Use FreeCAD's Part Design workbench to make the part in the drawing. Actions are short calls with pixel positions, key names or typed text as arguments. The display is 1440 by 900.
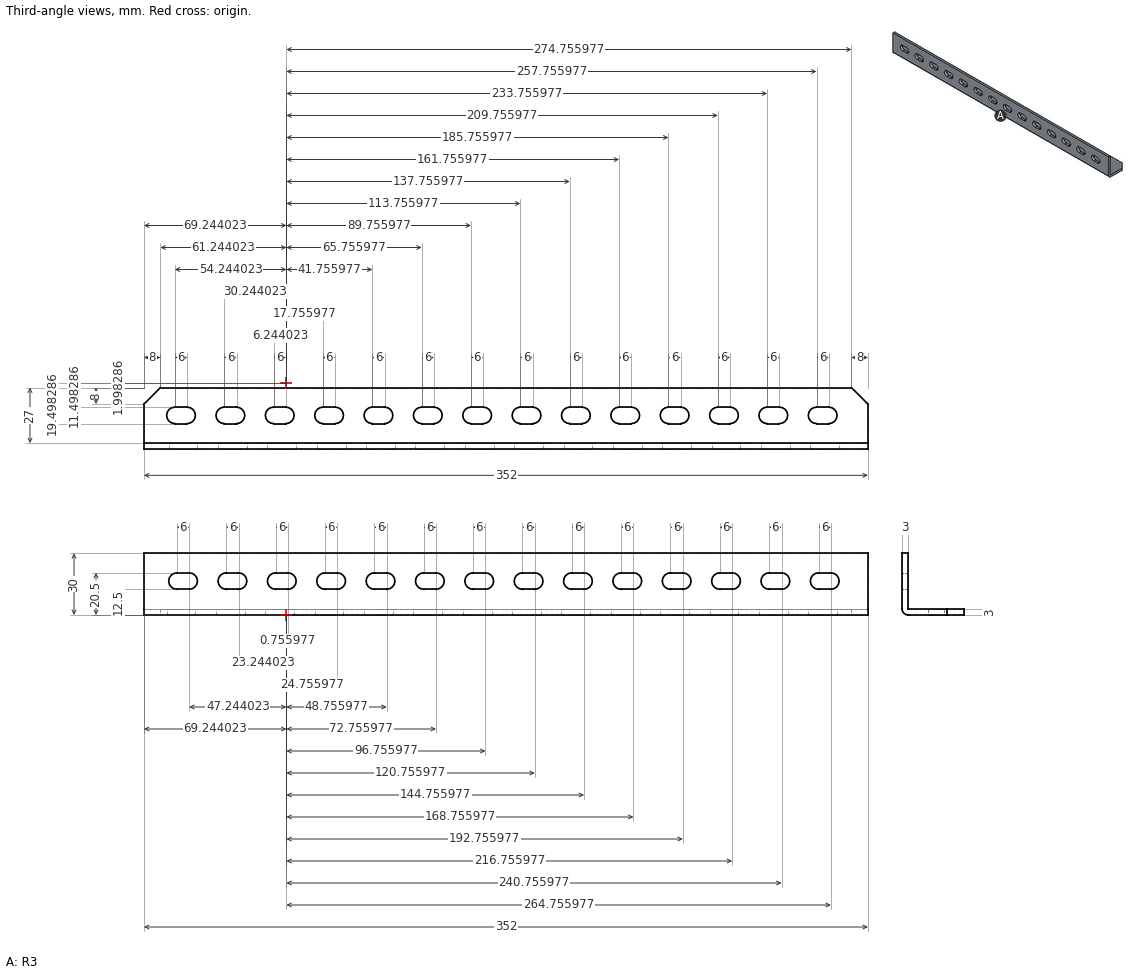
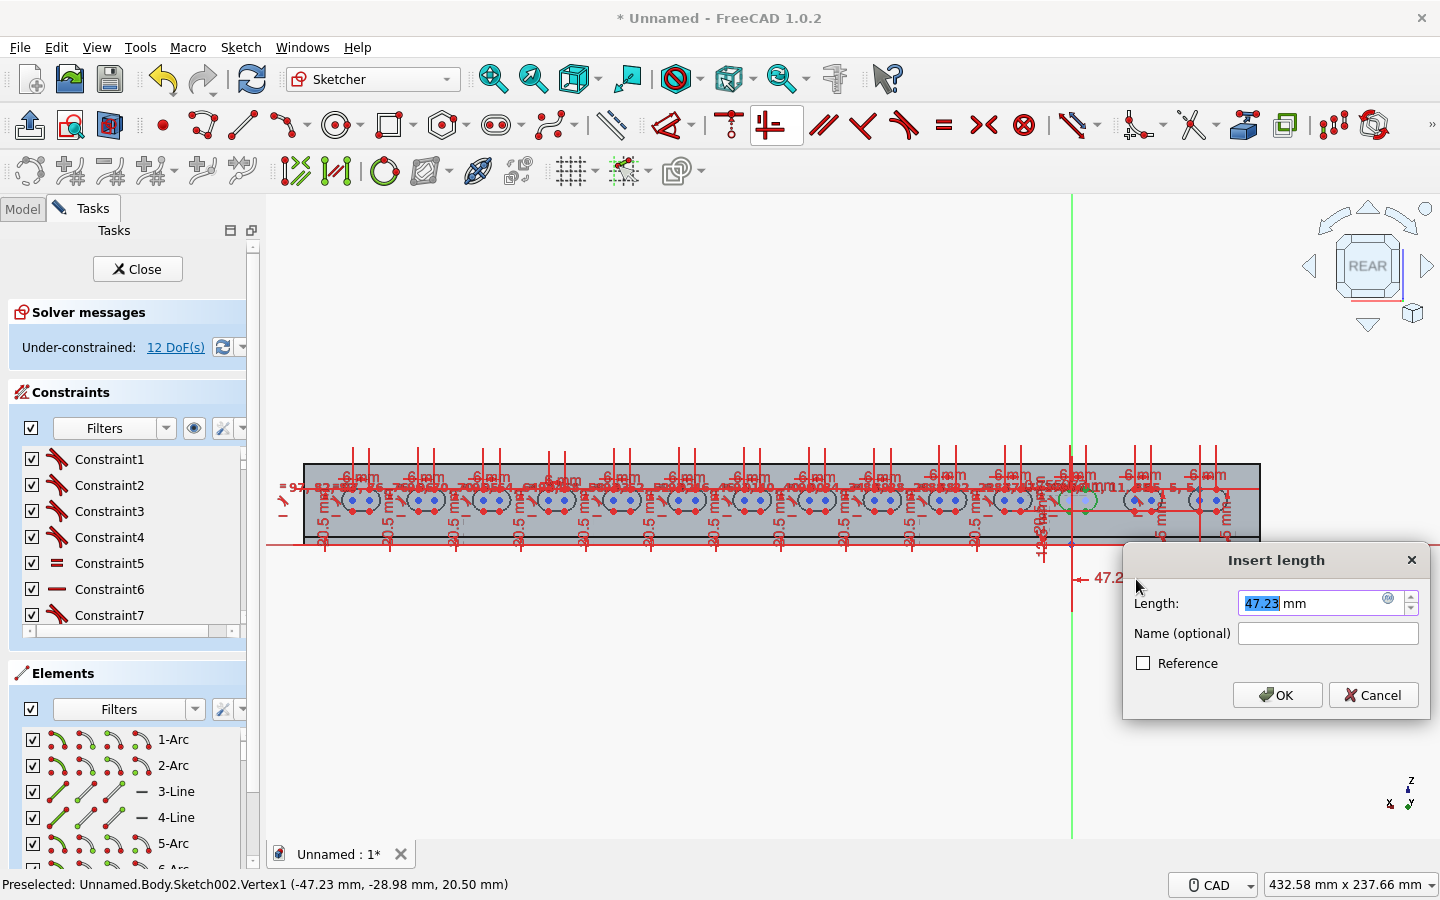
text(47.244023)
key(Return)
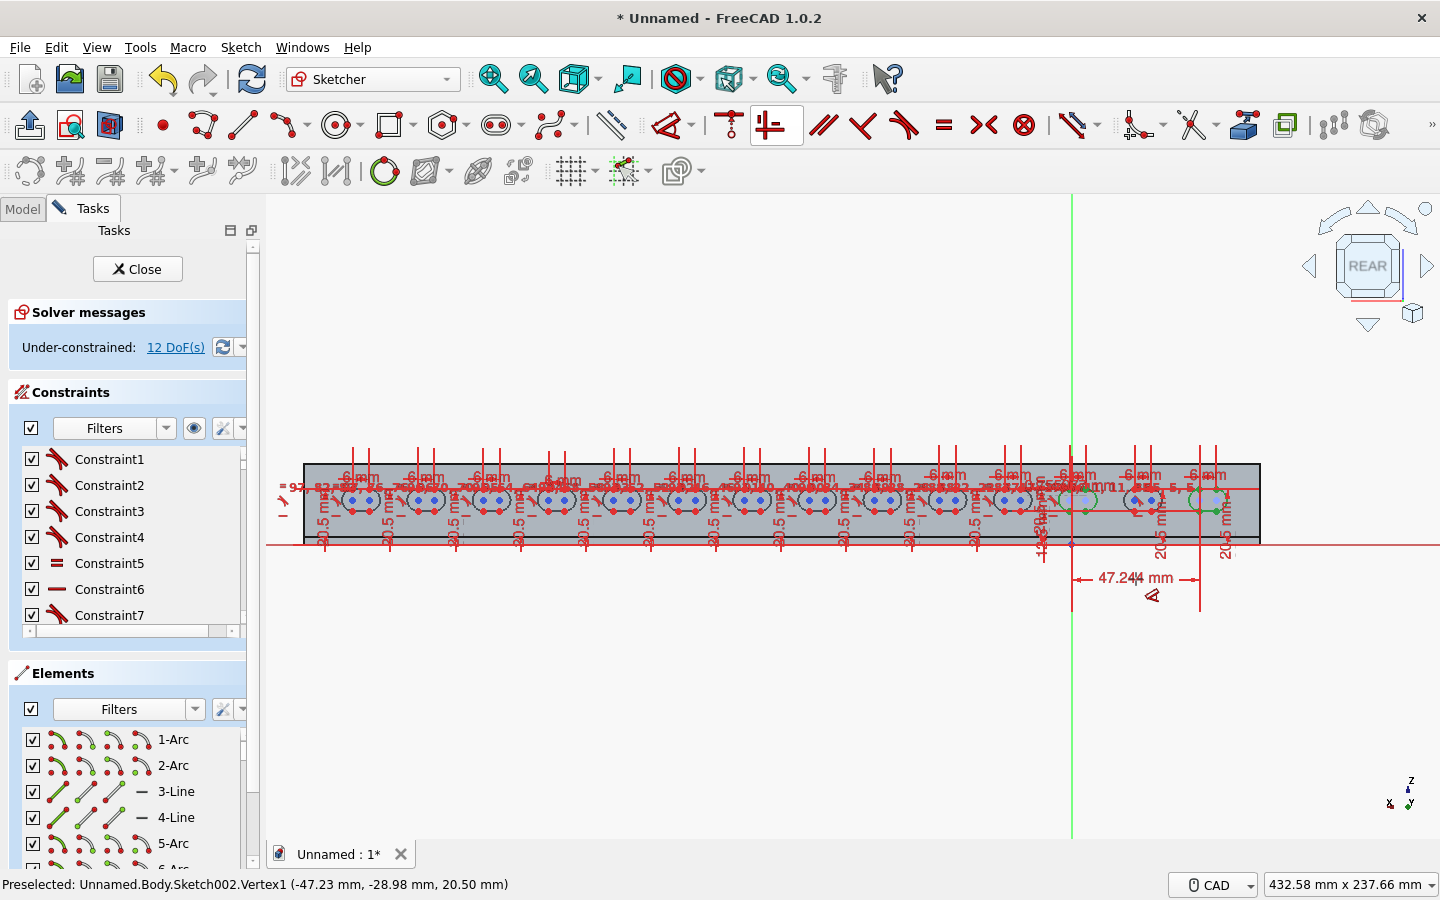
click(1135, 489)
click(1103, 455)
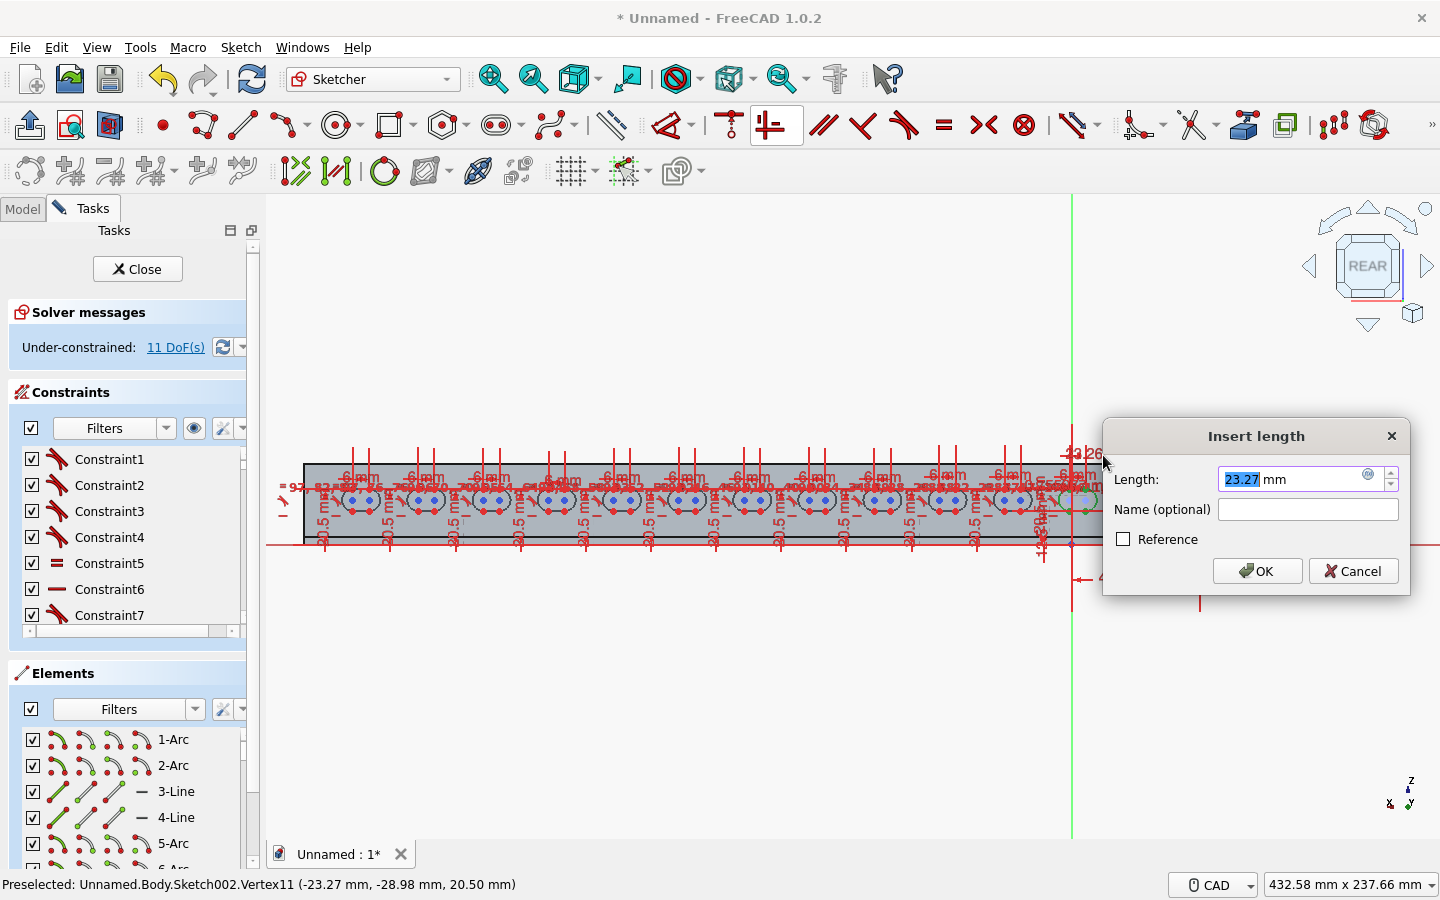
text(23.244023)
key(Return)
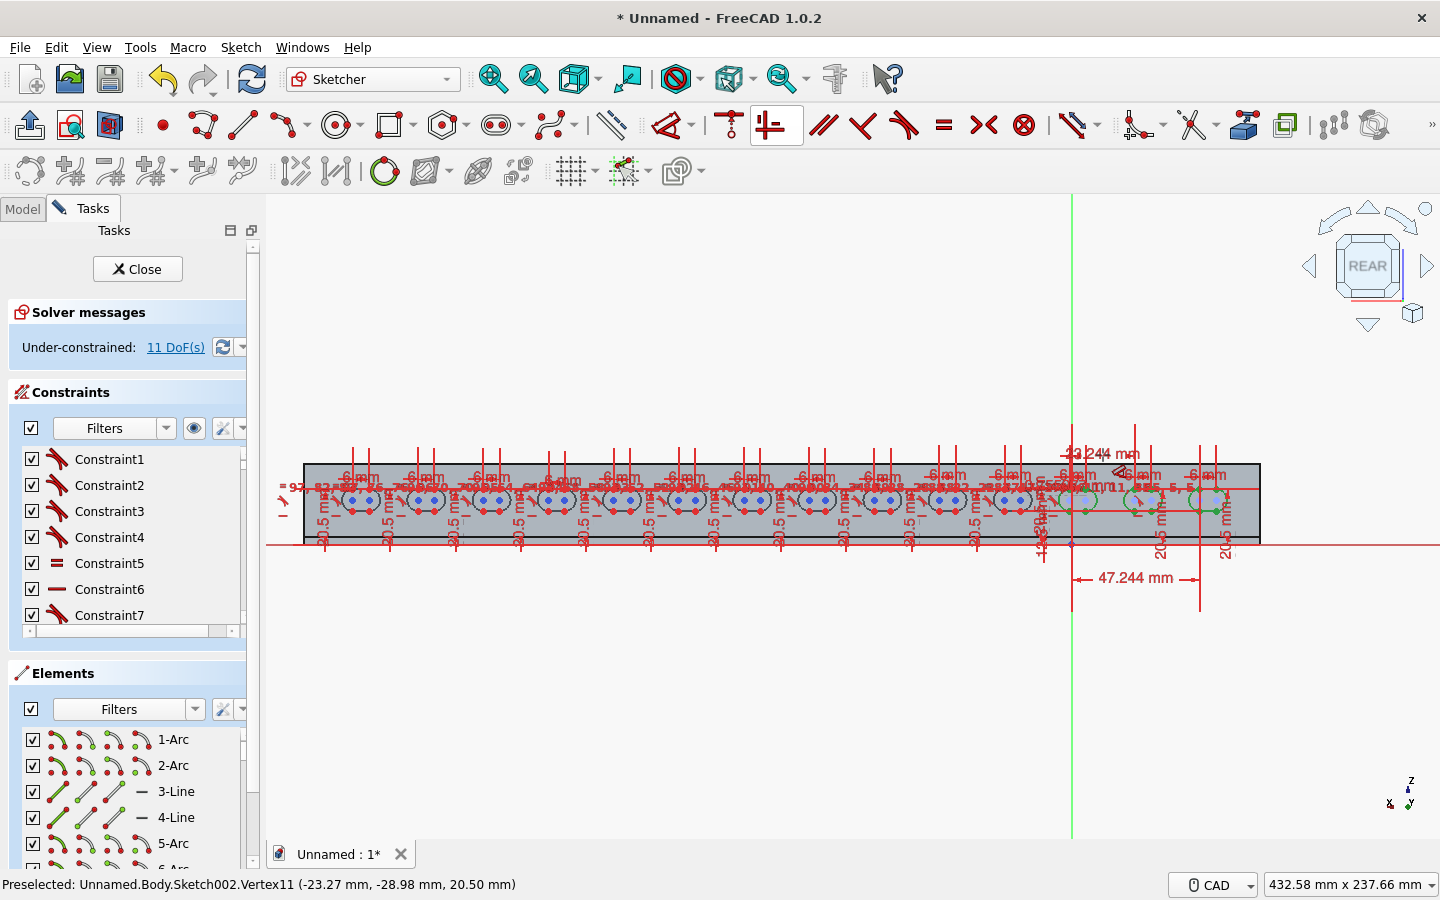
click(1005, 489)
click(1038, 579)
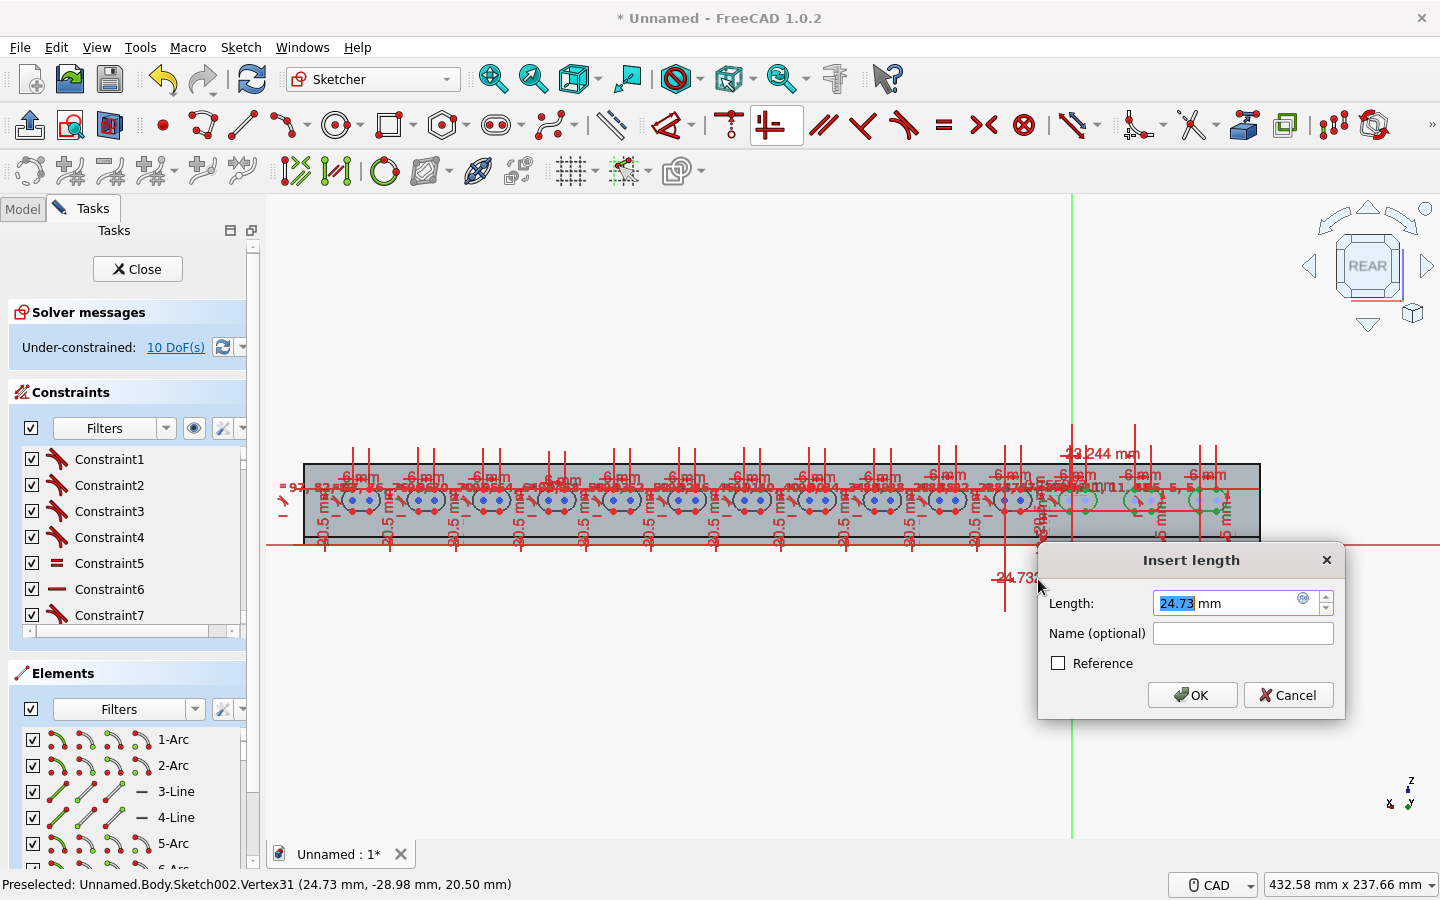
text(24.755977)
key(Return)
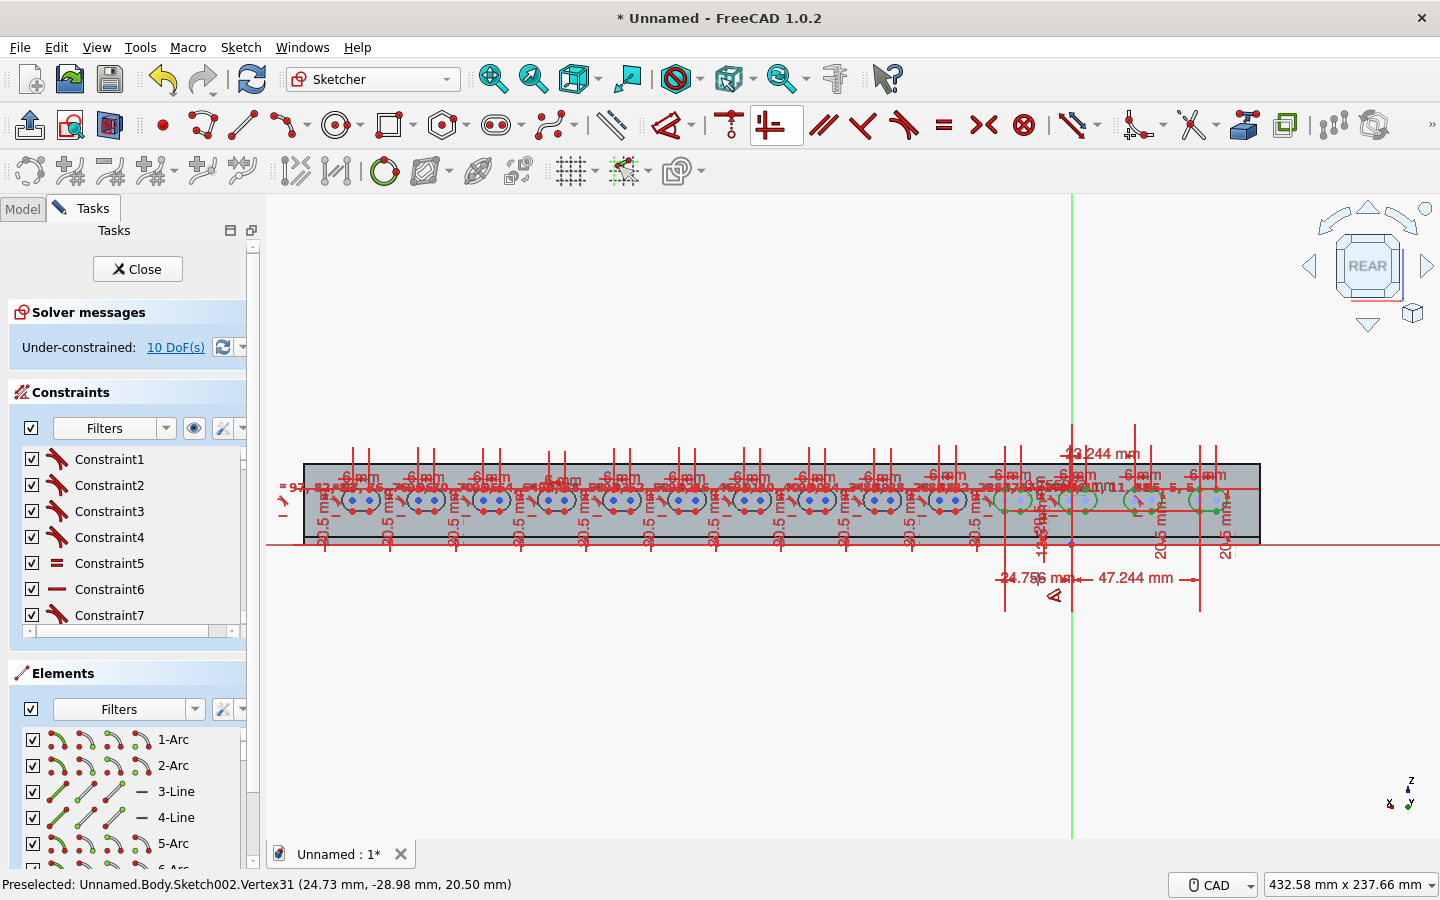
click(939, 489)
click(959, 579)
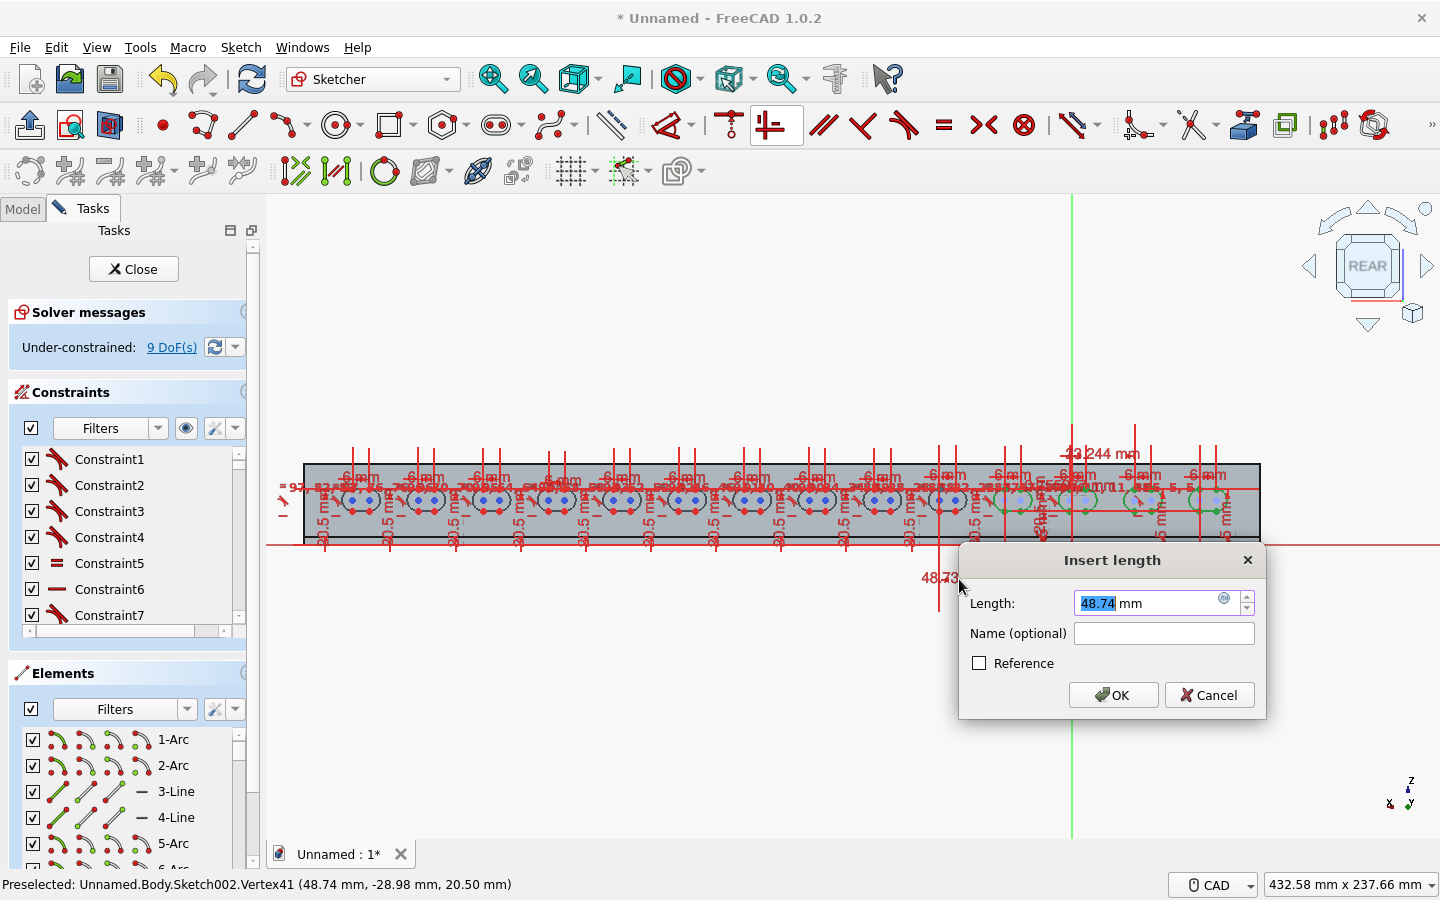
text(48.755977)
key(Return)